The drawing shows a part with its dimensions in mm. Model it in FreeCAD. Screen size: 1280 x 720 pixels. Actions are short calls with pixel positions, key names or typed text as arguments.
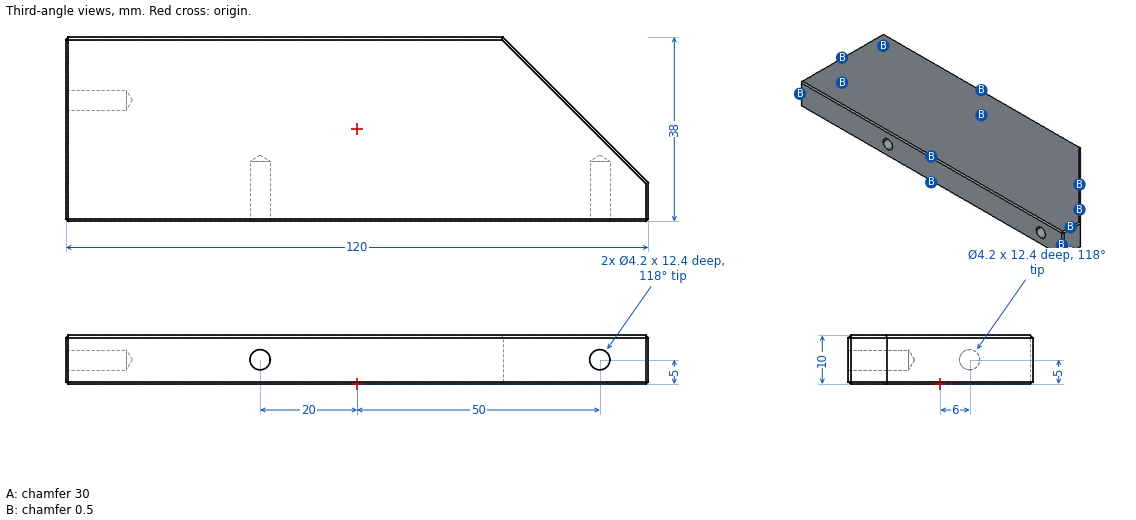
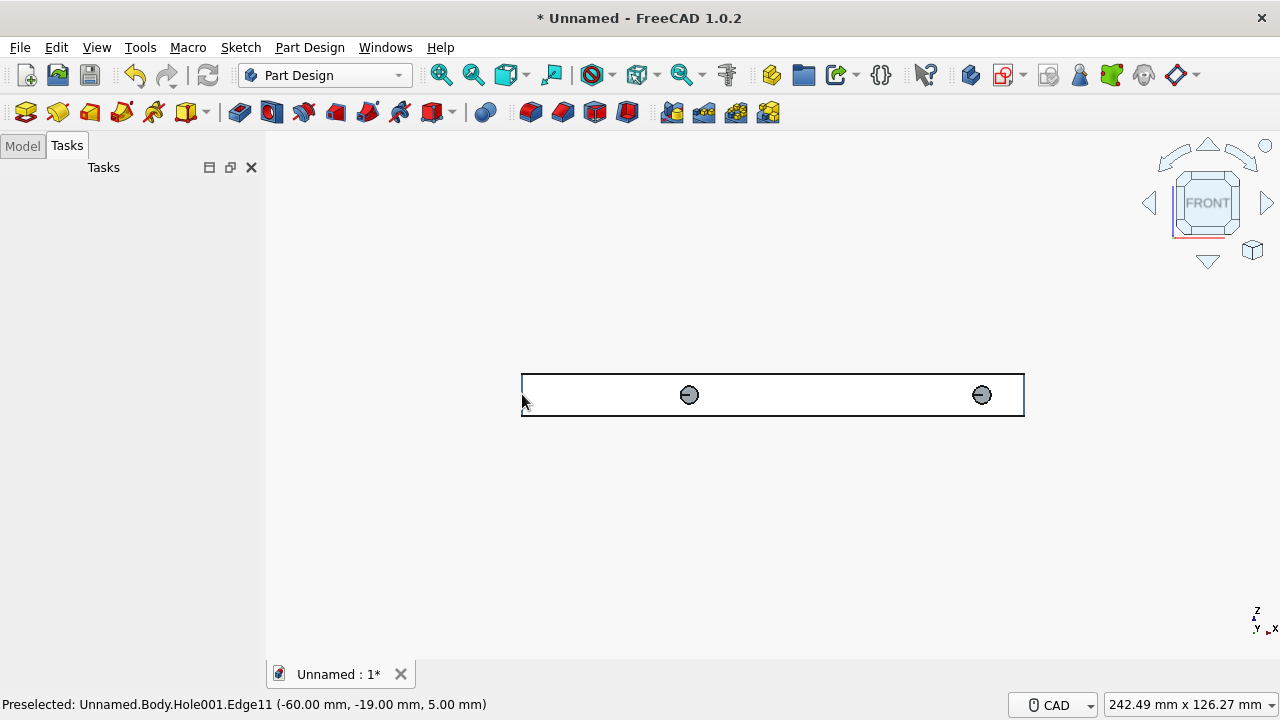
key(3)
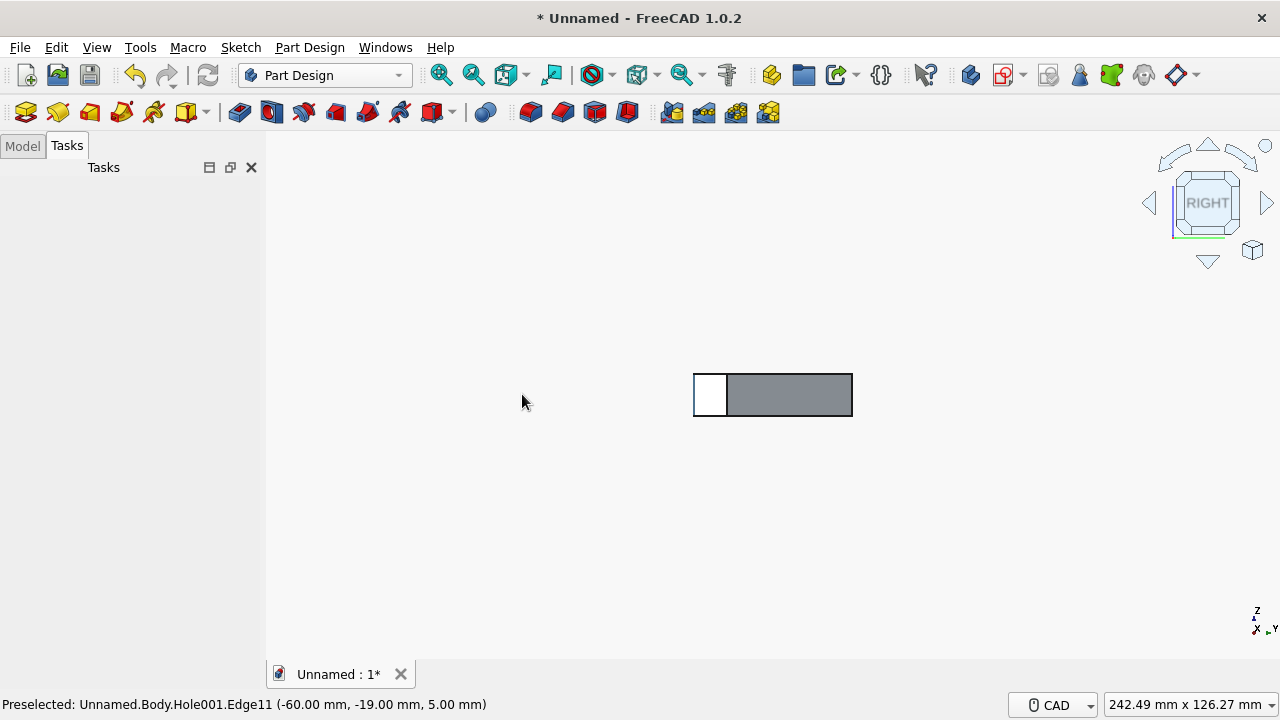
click(442, 76)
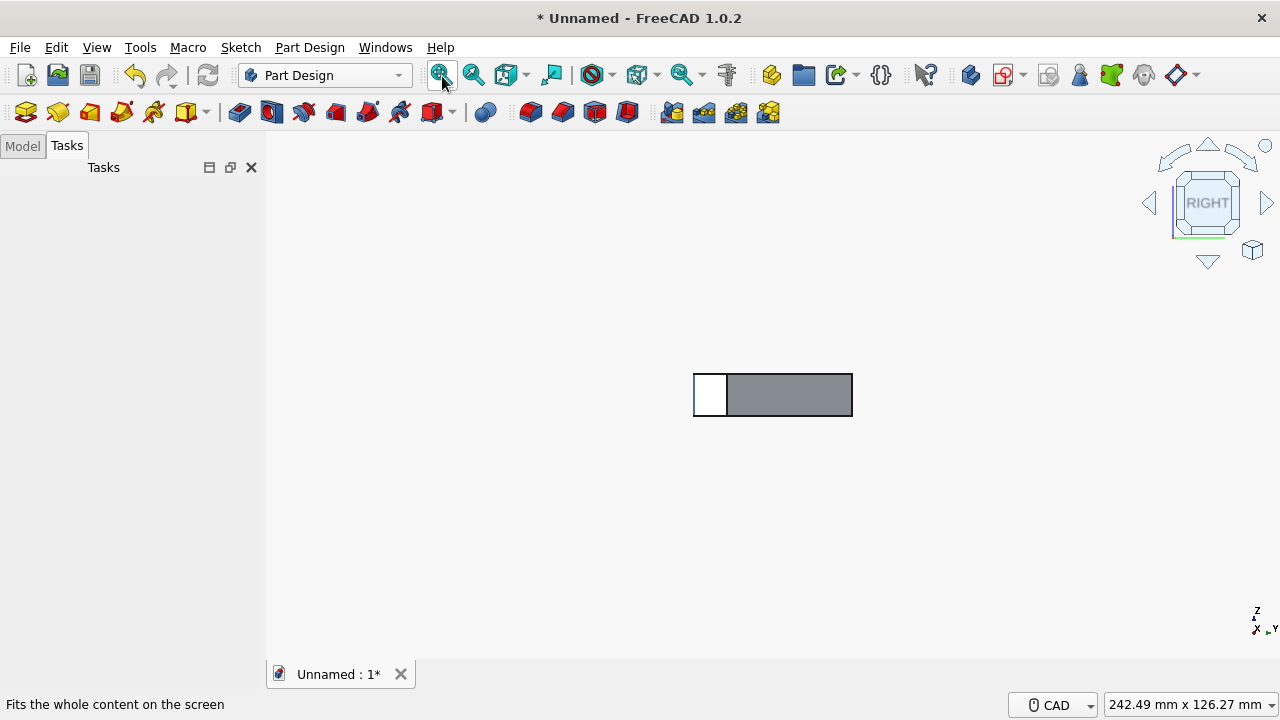
key(5)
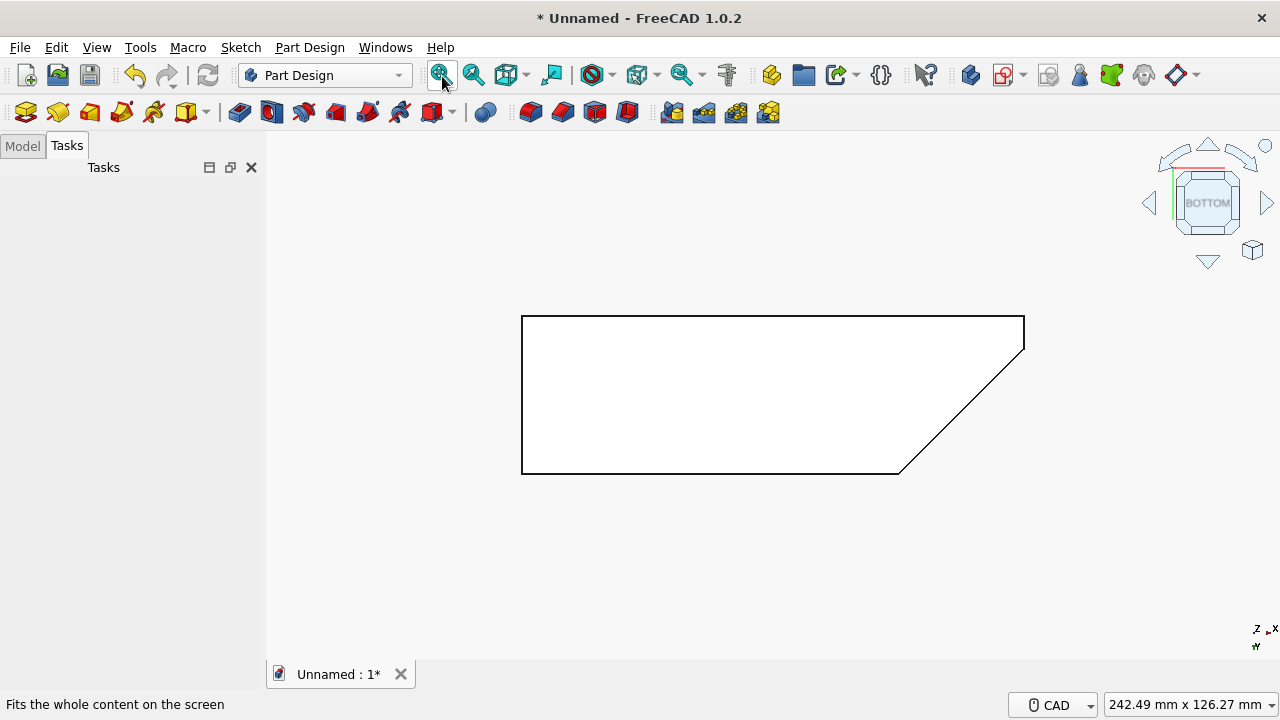
click(845, 394, ctrl)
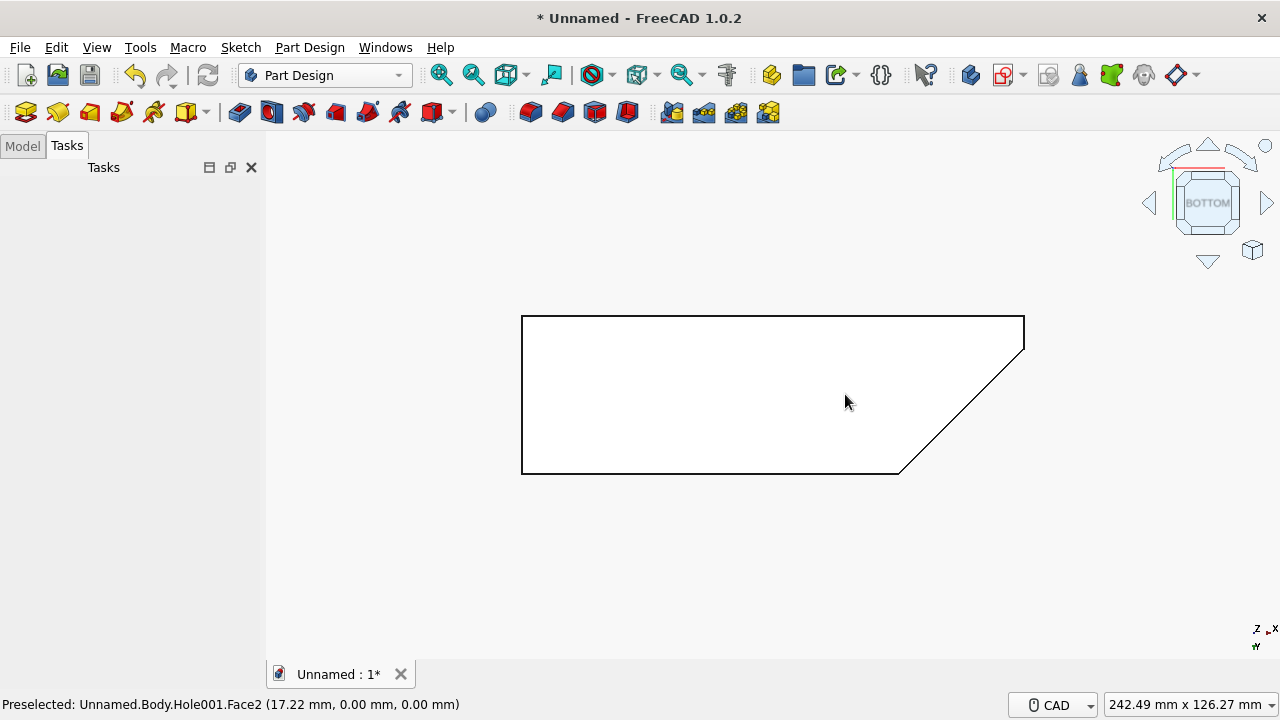
key(4)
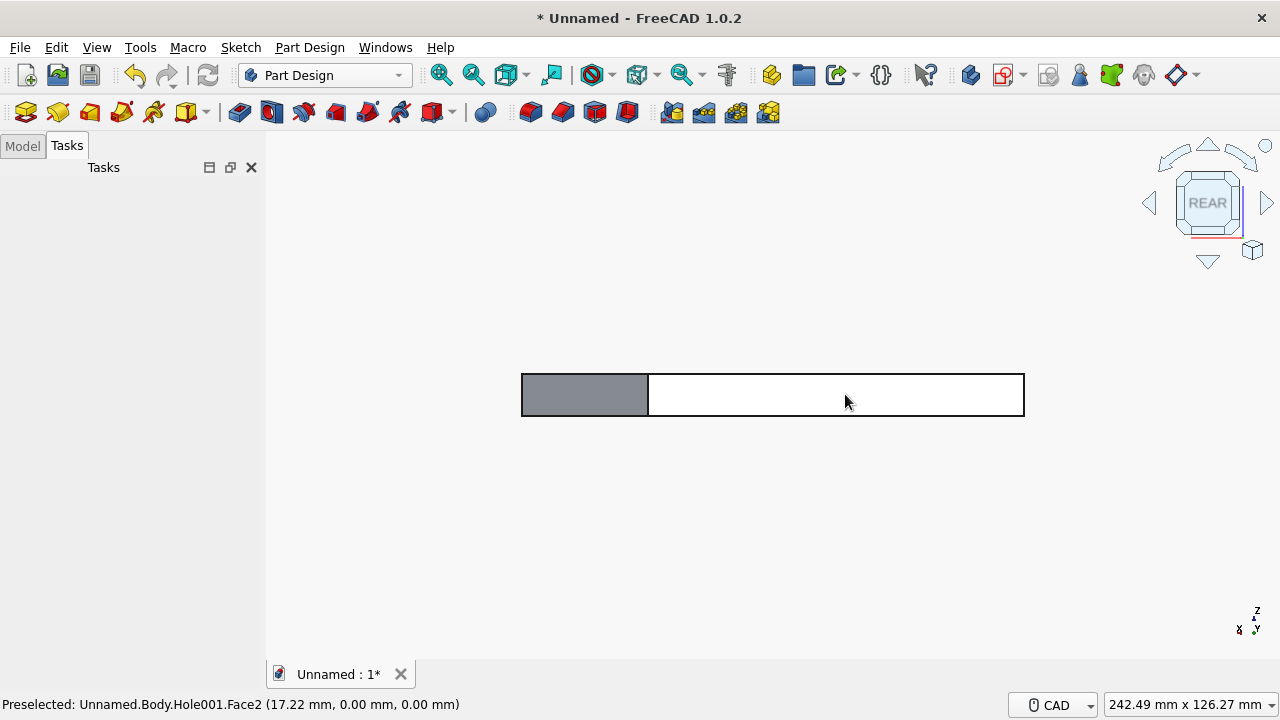
click(1024, 394, ctrl)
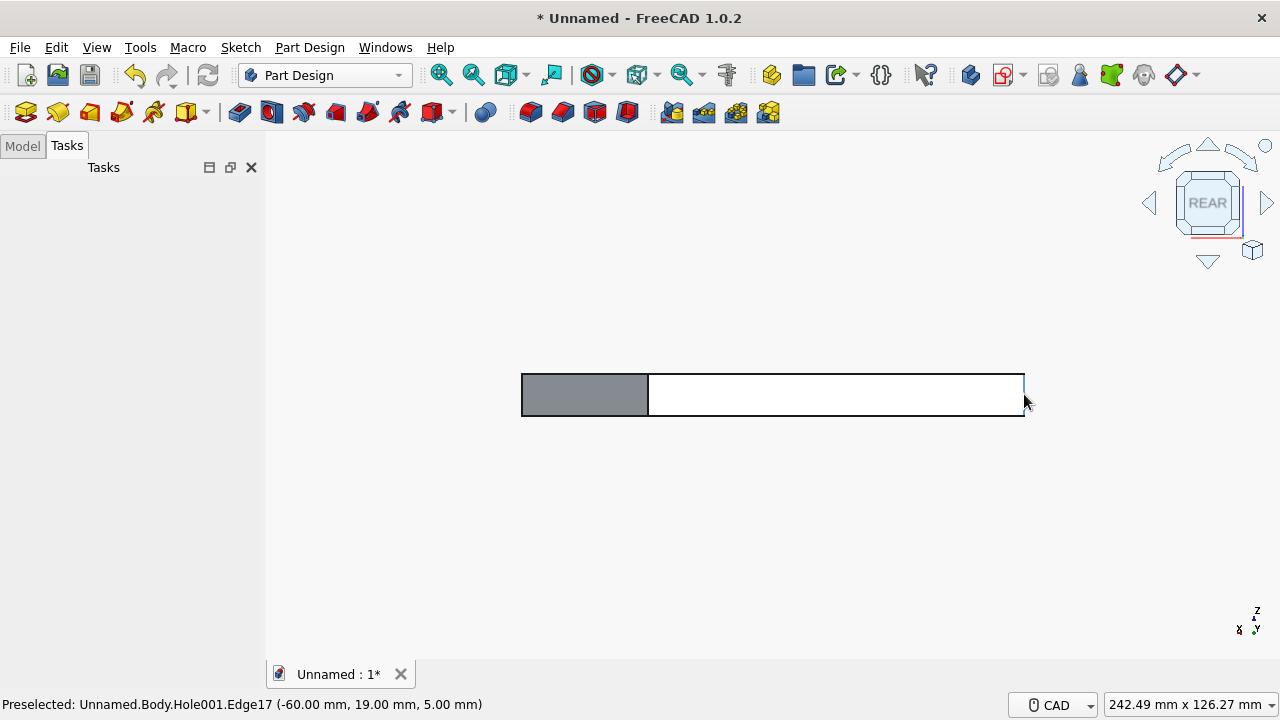
click(564, 112)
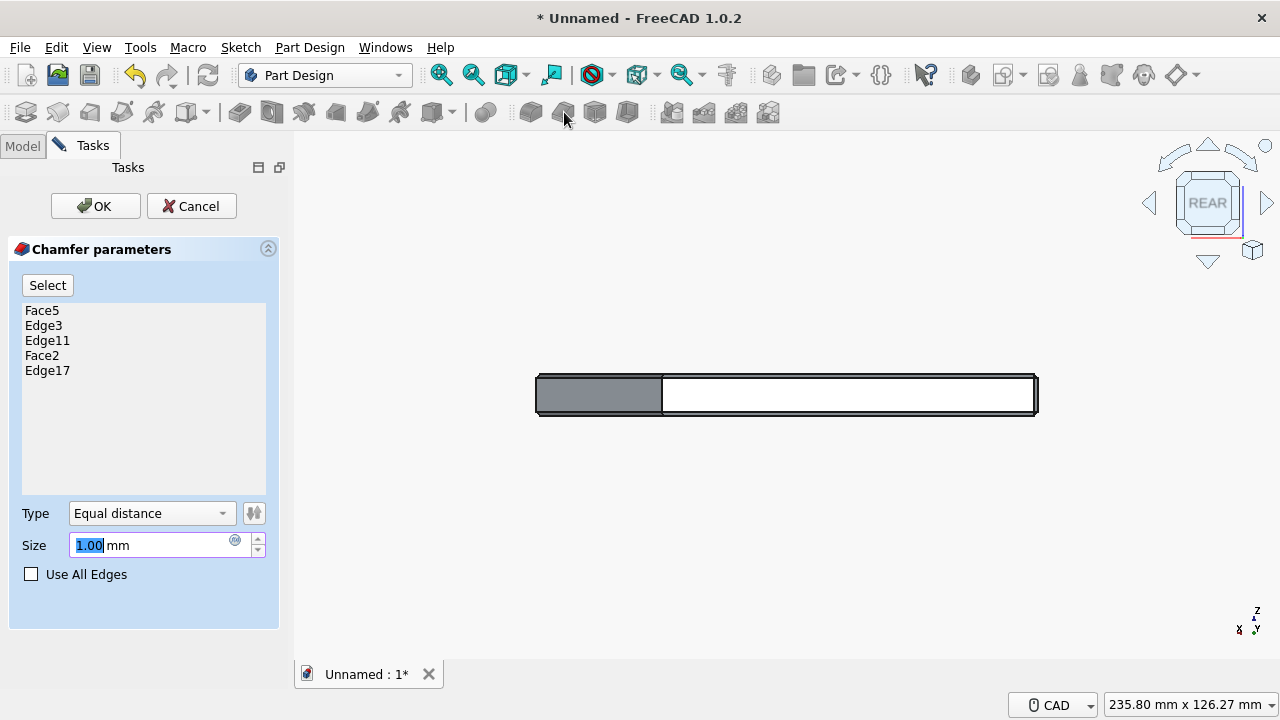
text(0.5)
key(Tab)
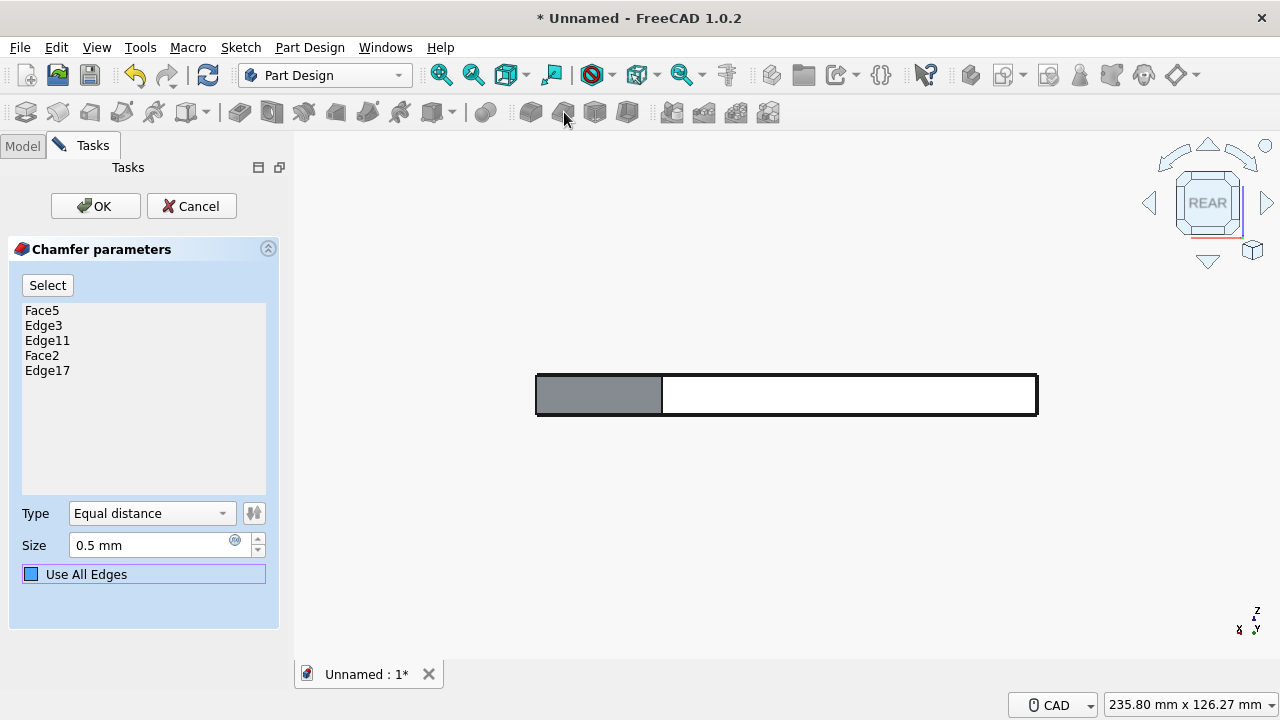
click(96, 206)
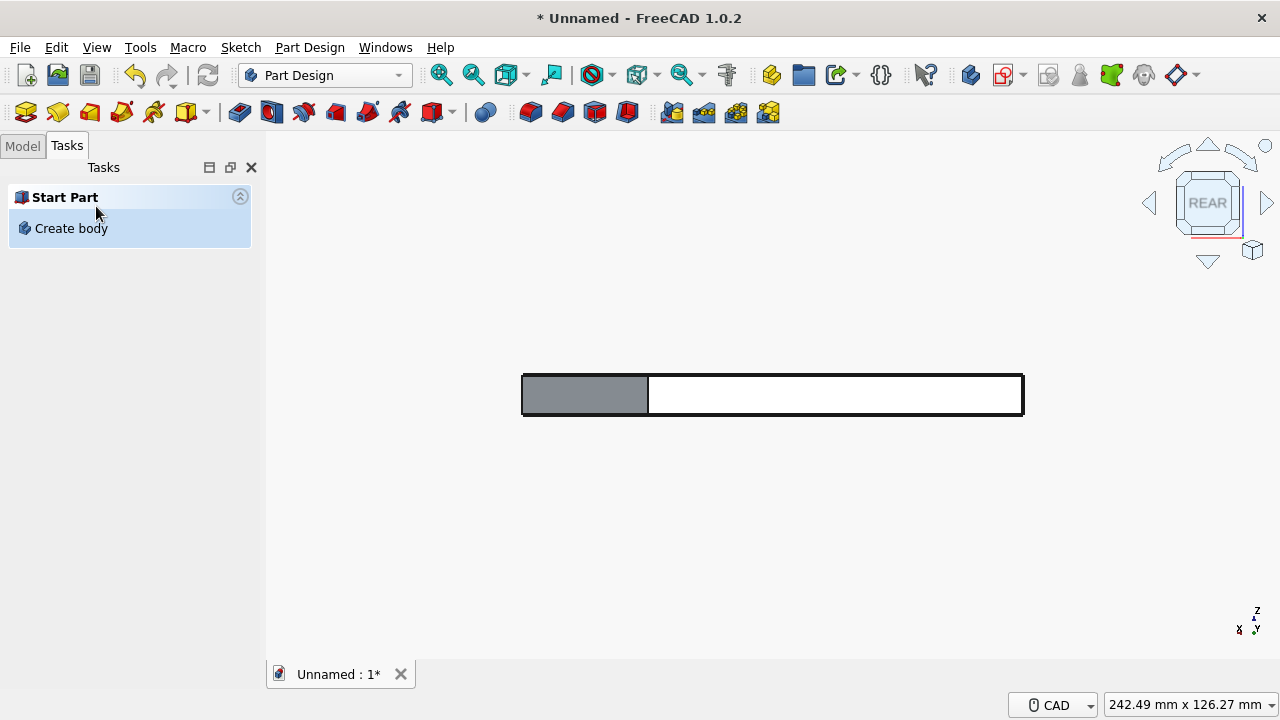
key(0)